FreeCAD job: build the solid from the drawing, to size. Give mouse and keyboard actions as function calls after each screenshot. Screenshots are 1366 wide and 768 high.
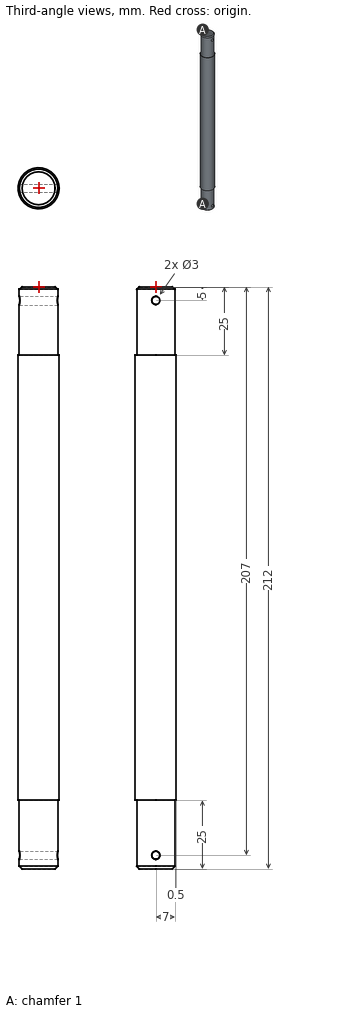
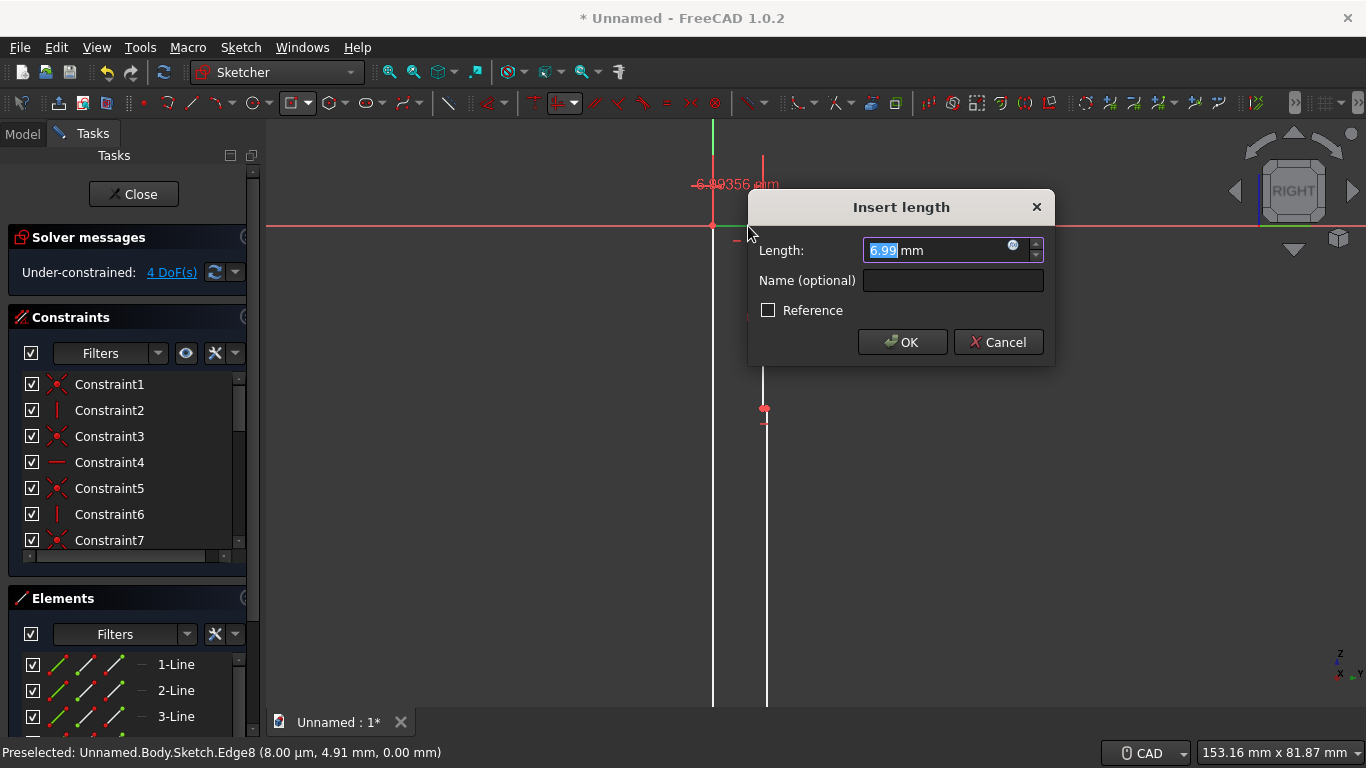
text(7)
key(Return)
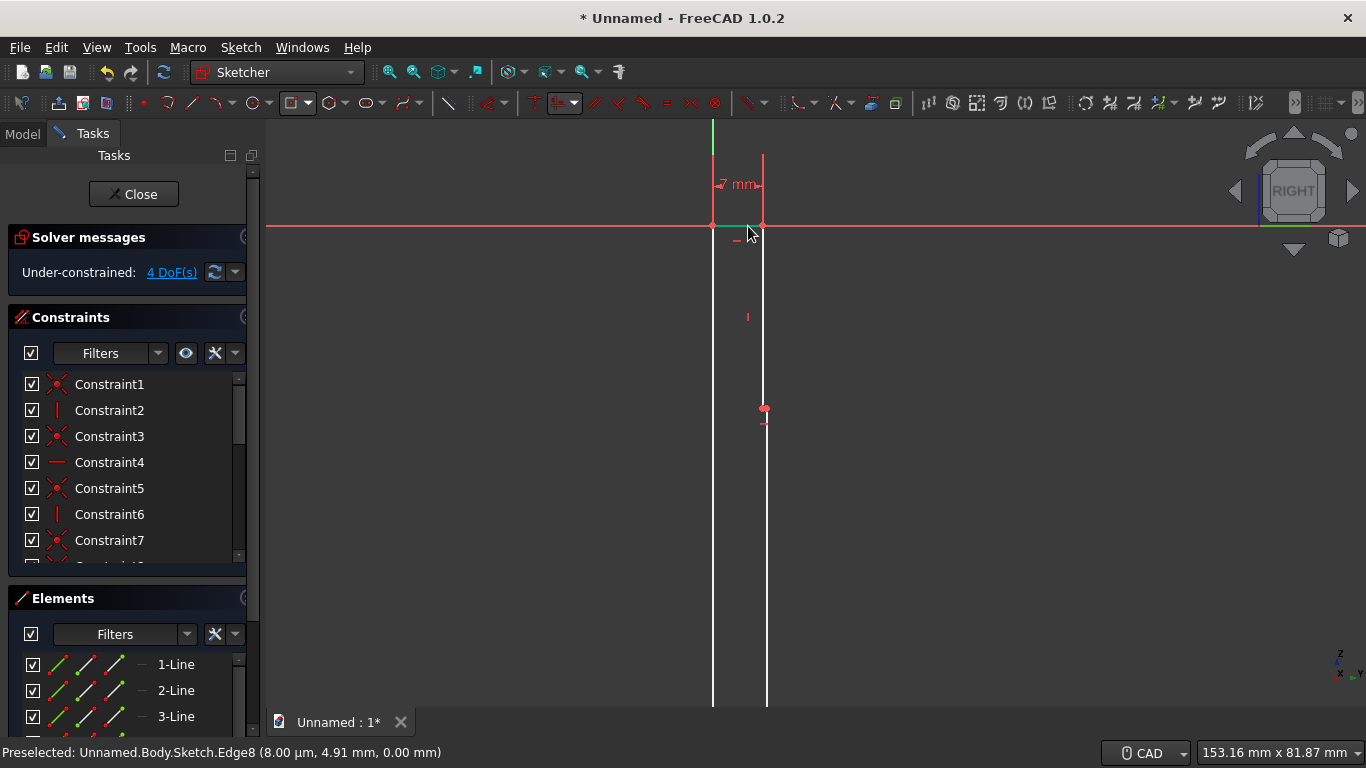
scroll(750, 225, down, 7)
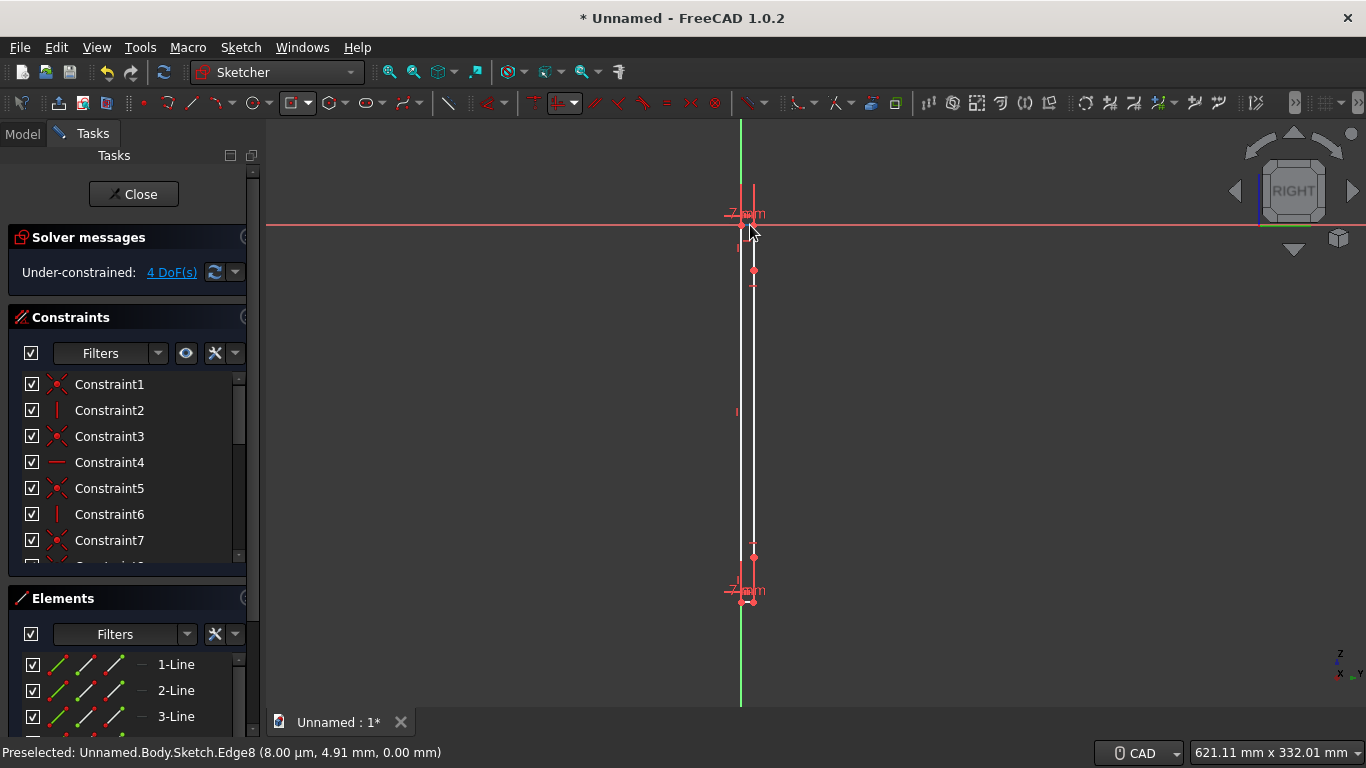
click(754, 571)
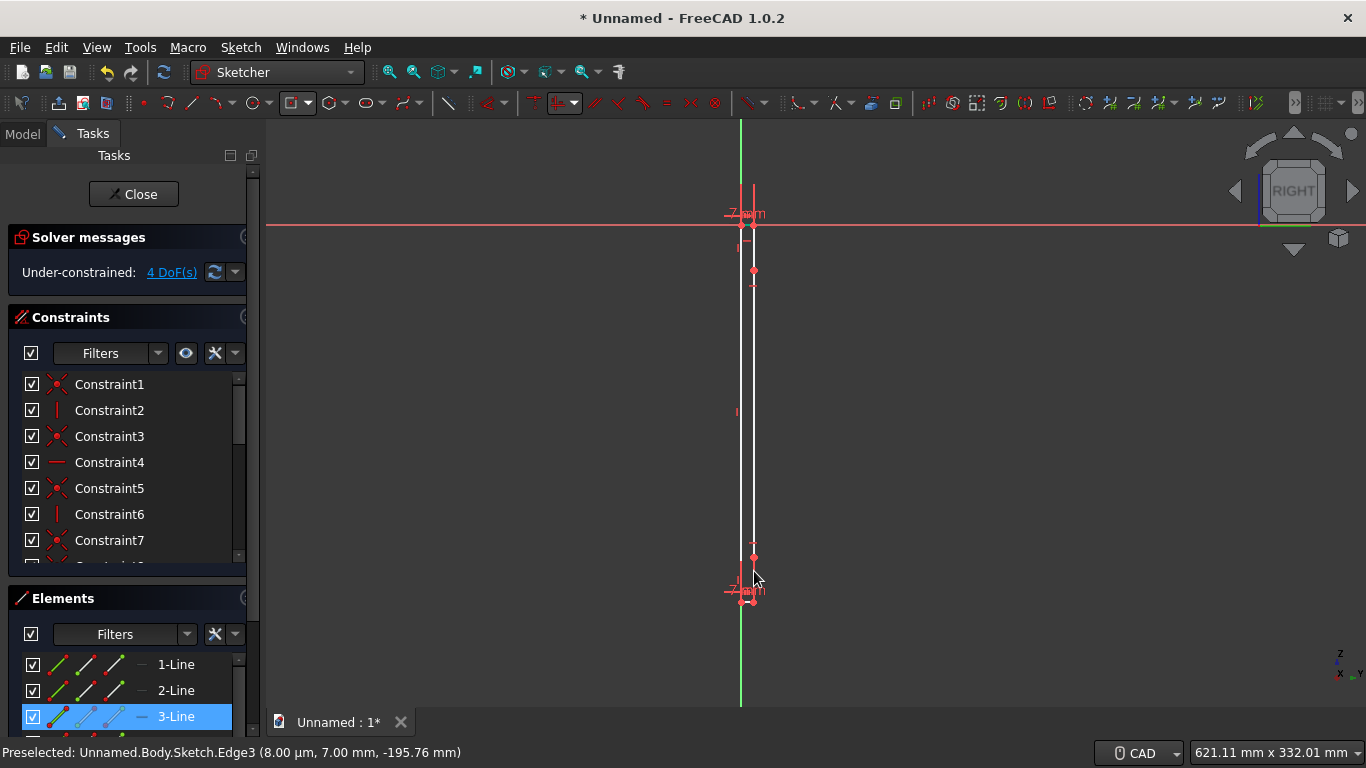
key(i)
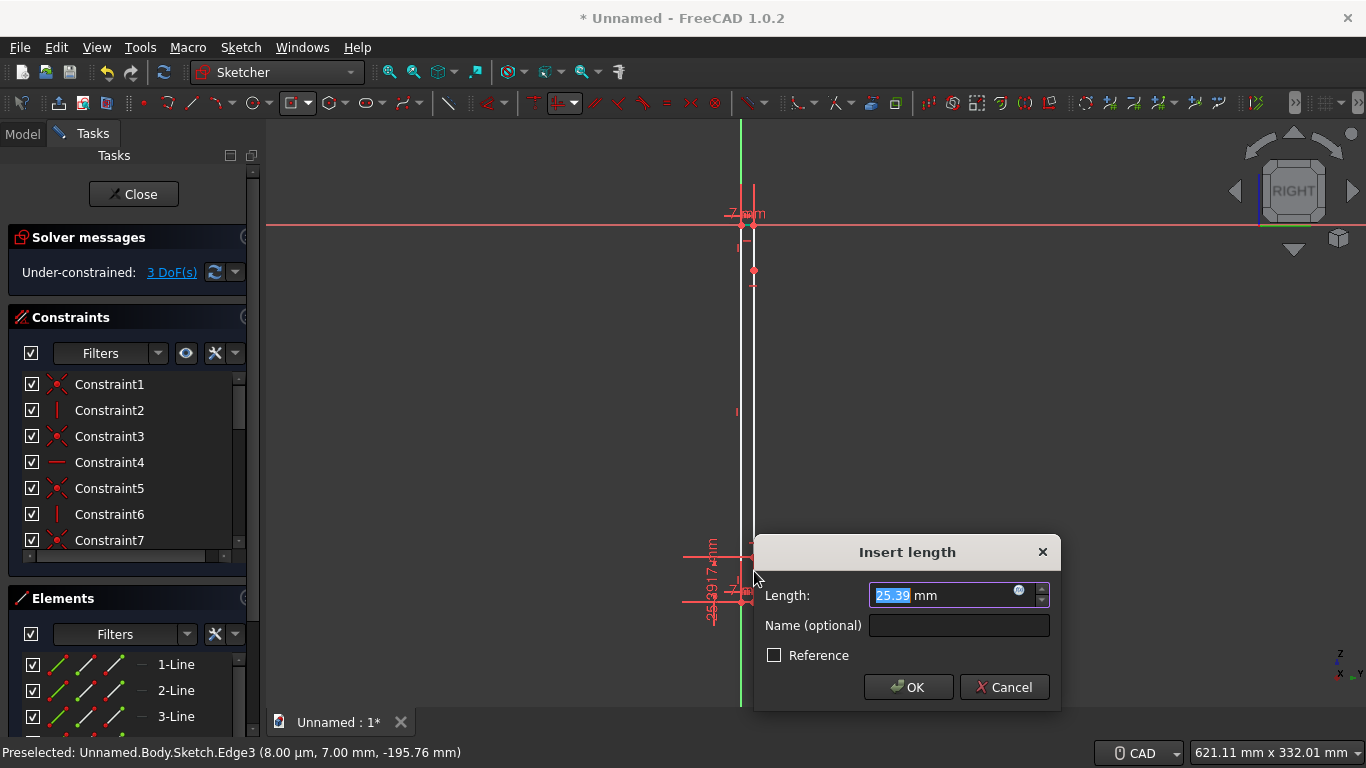
text(25)
key(Return)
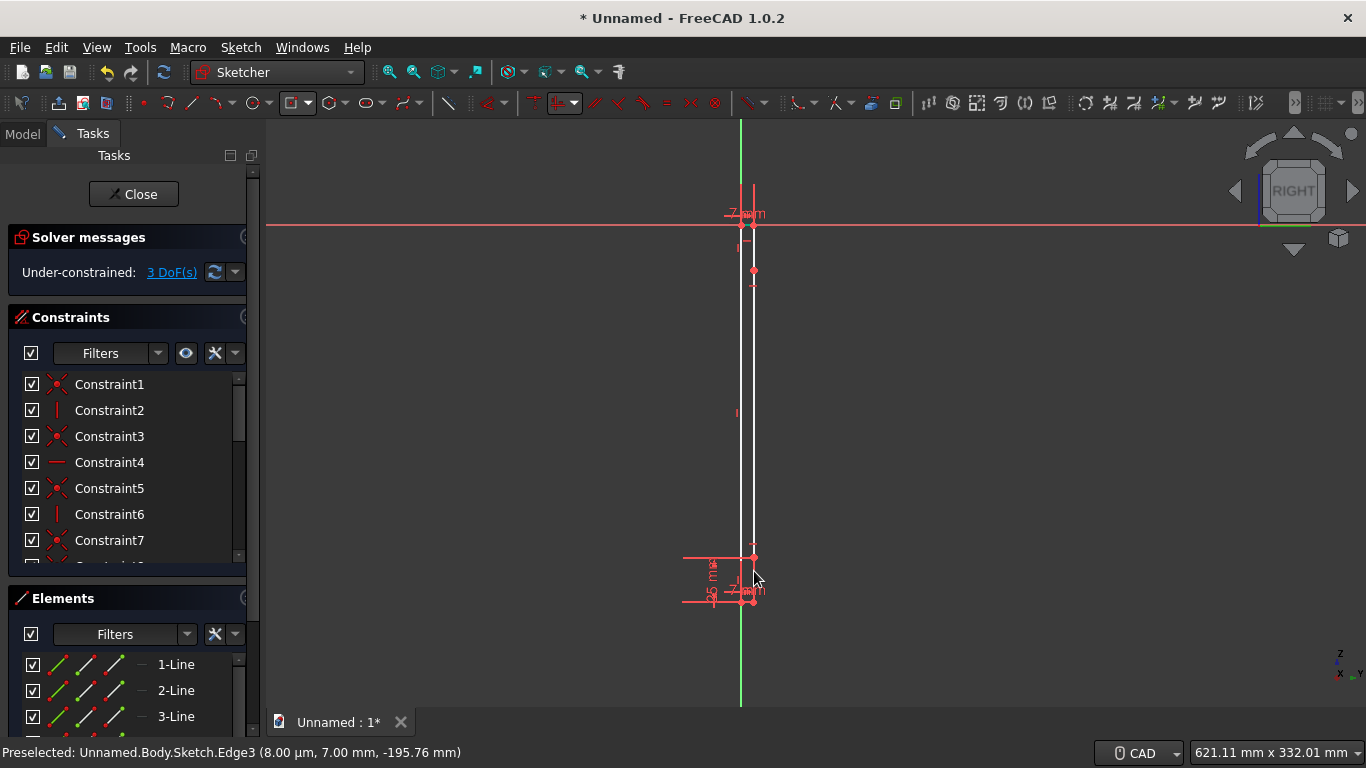
click(754, 257)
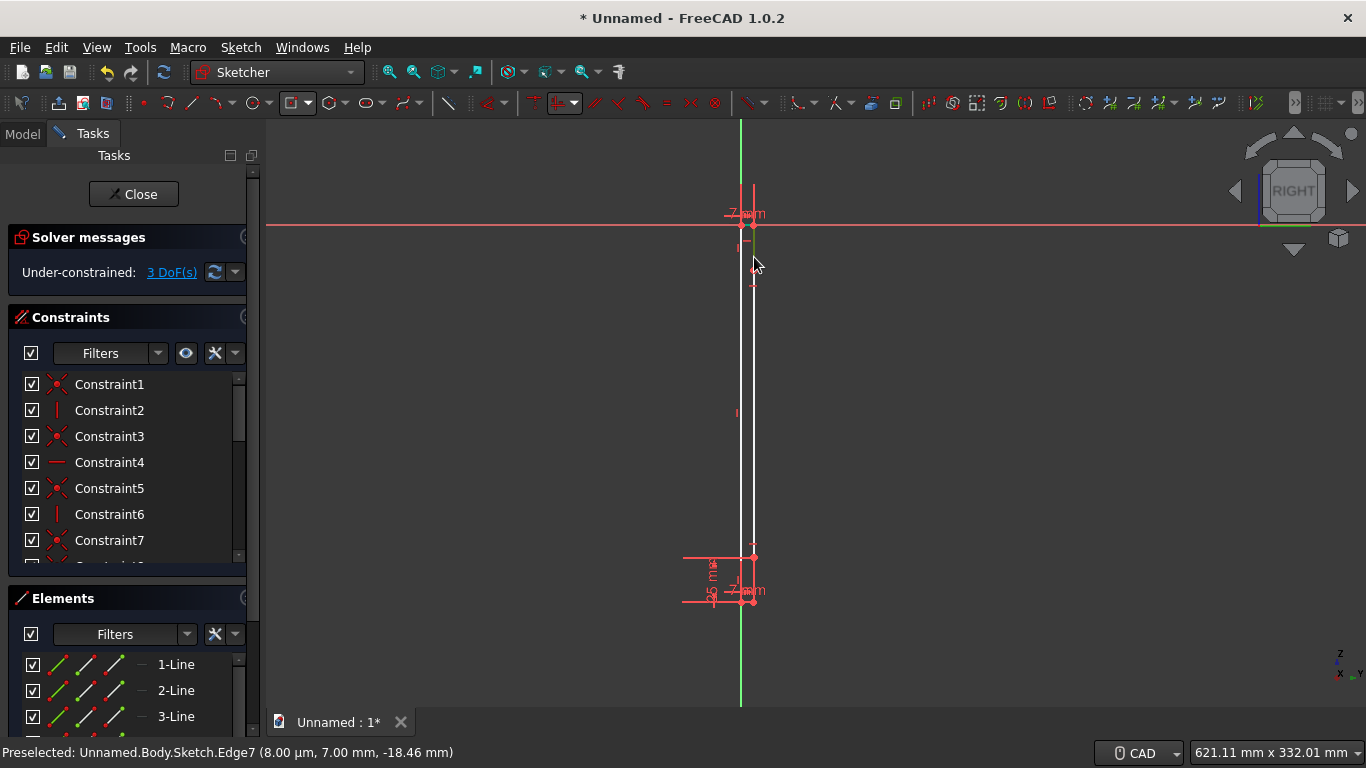
key(i)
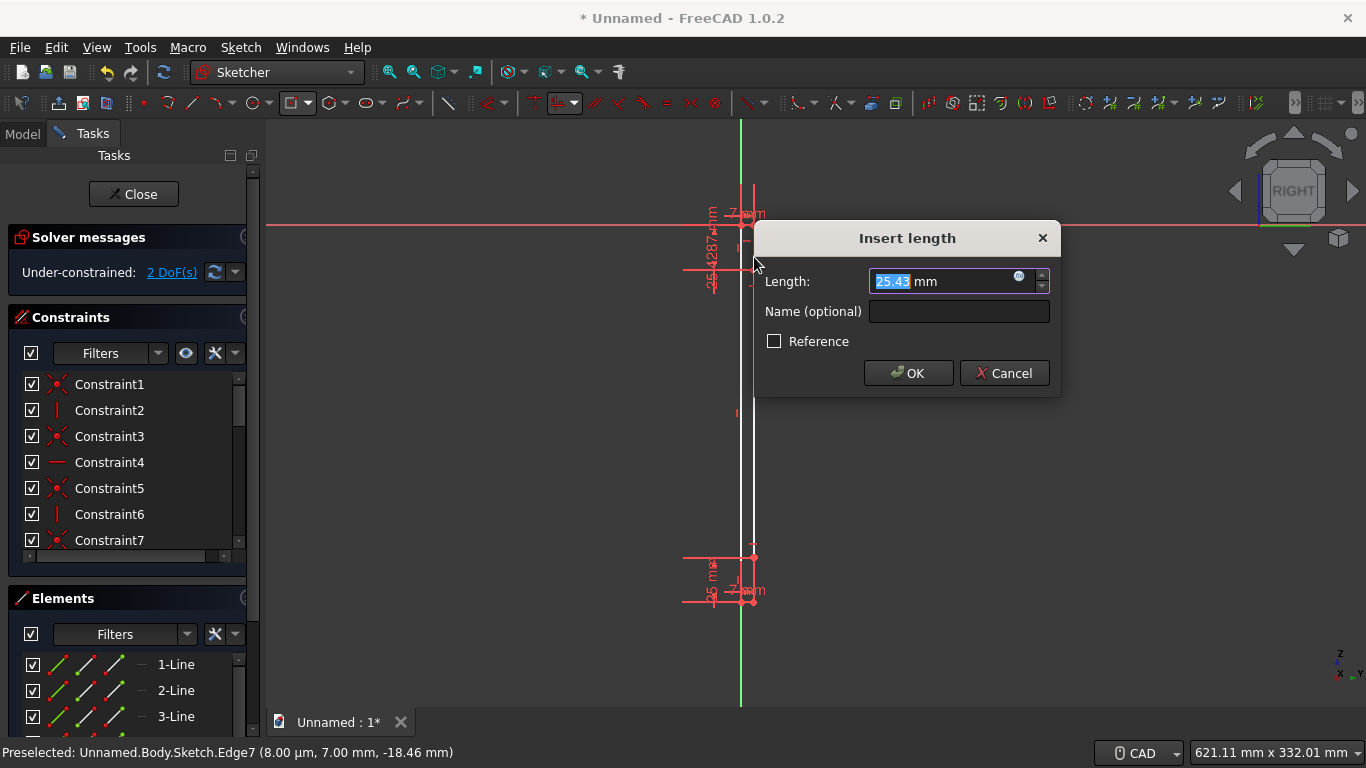
text(25)
key(Return)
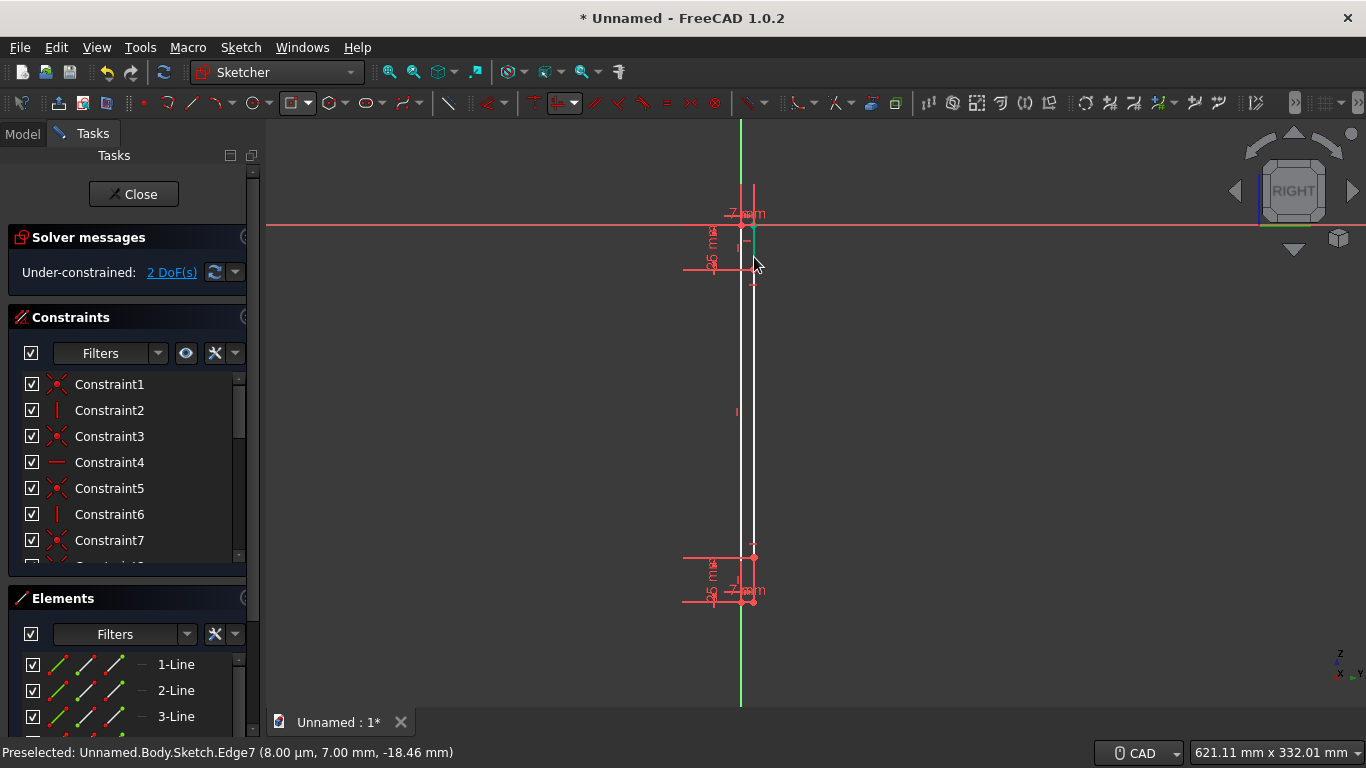
click(741, 338)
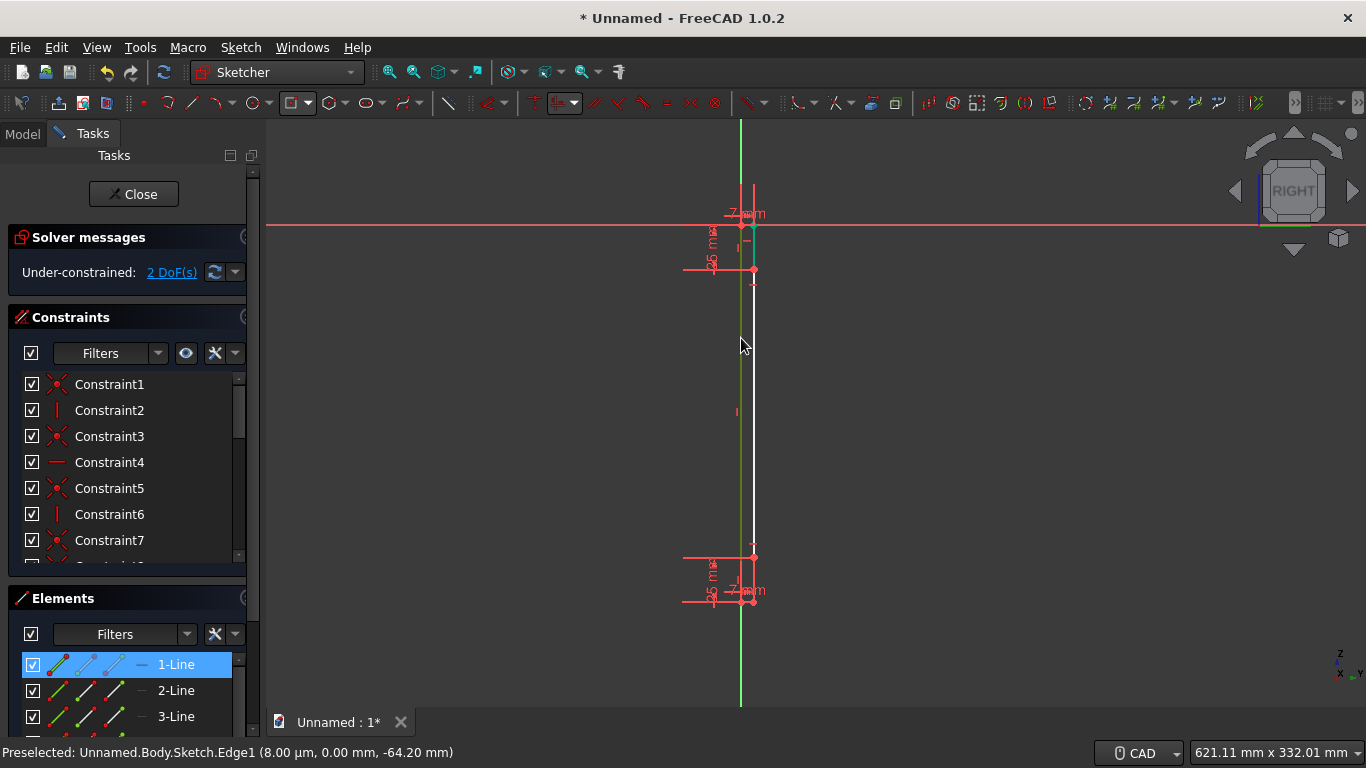
key(i)